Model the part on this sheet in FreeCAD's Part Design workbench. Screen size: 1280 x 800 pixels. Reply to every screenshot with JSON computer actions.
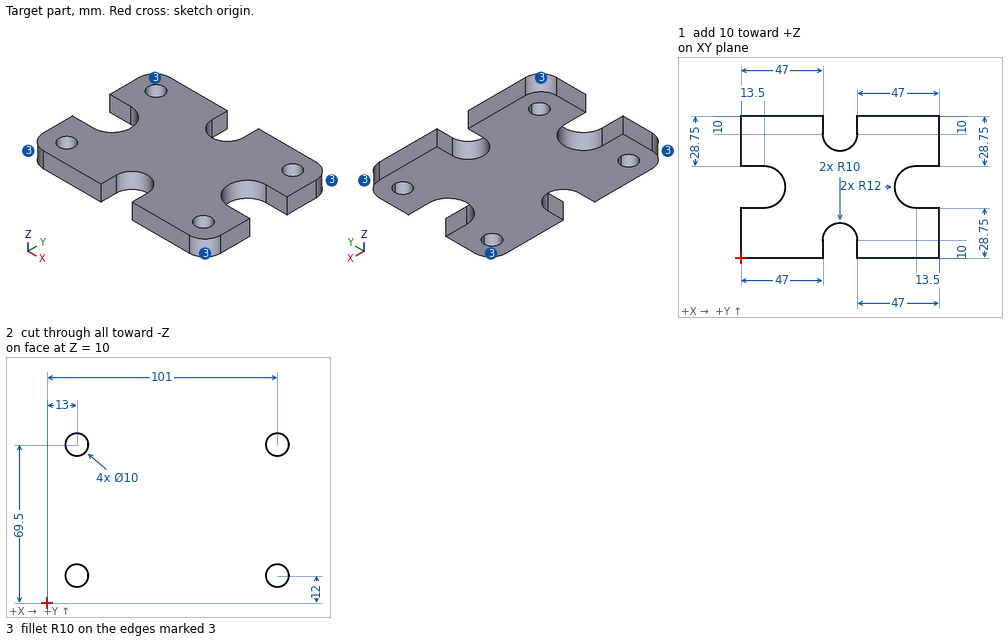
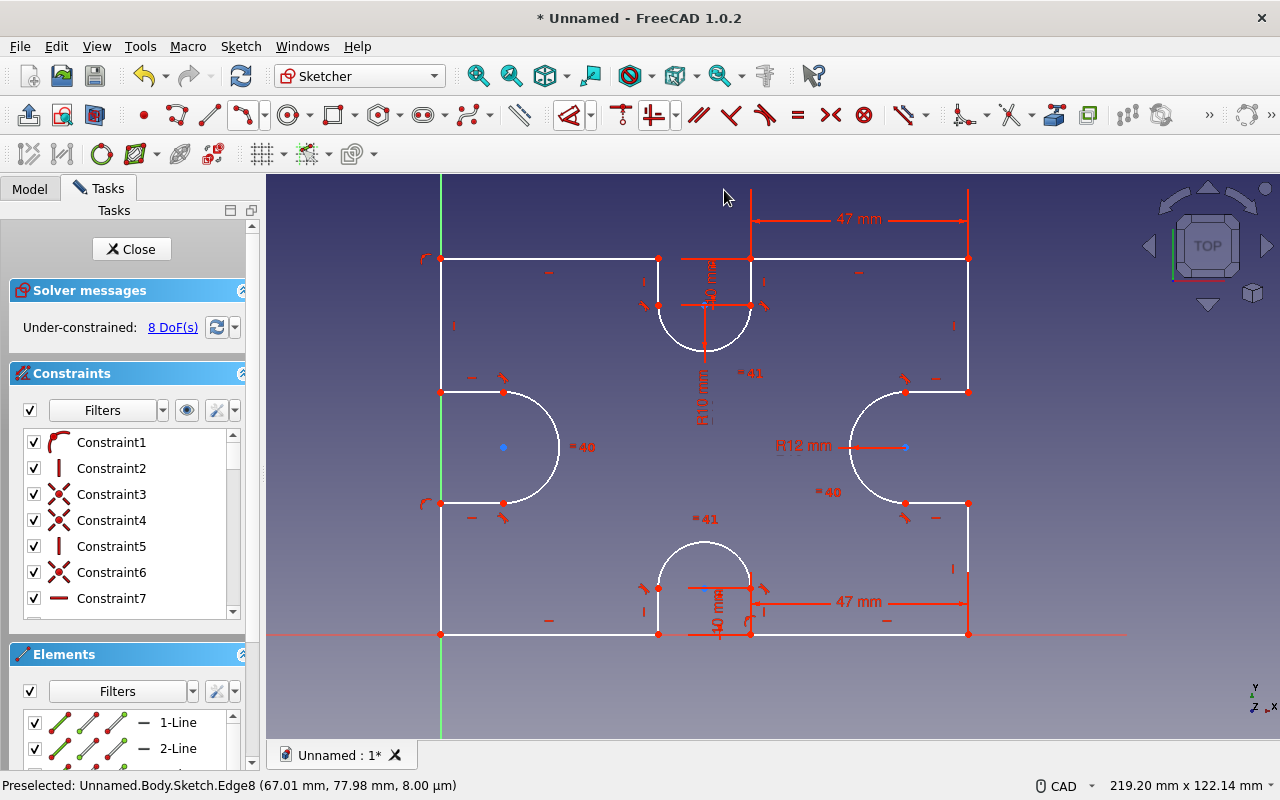
{"action": "left_click", "coordinate": [658, 291]}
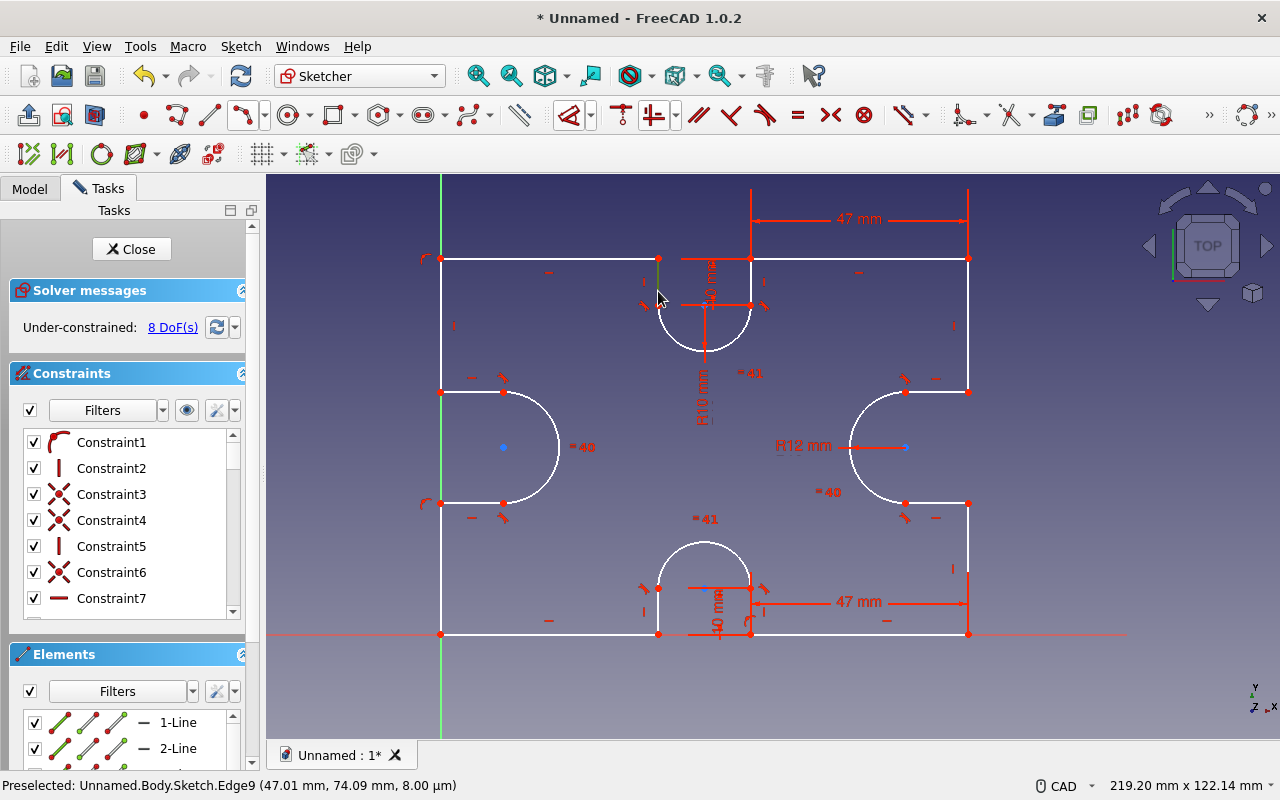
{"action": "key", "text": "i"}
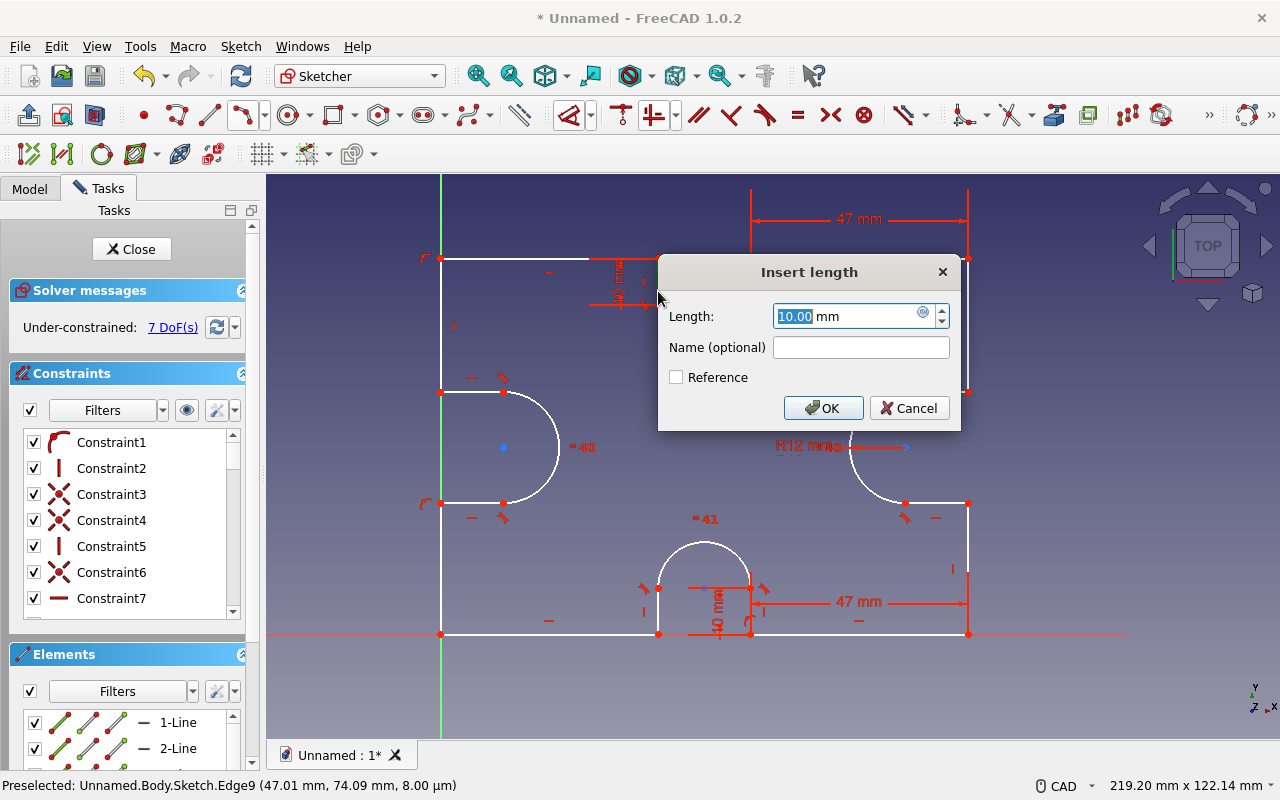
{"action": "type", "text": "10"}
{"action": "key", "text": "Return"}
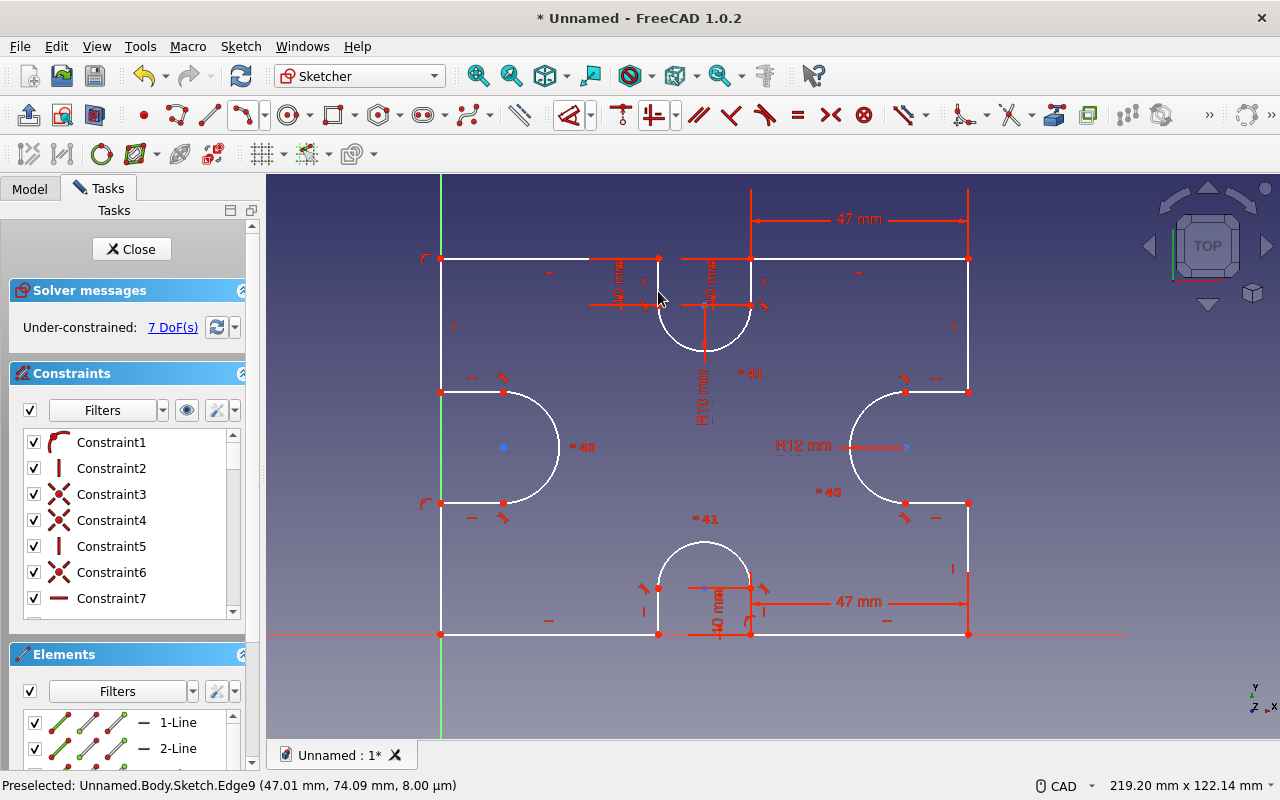
{"action": "left_click", "coordinate": [593, 259]}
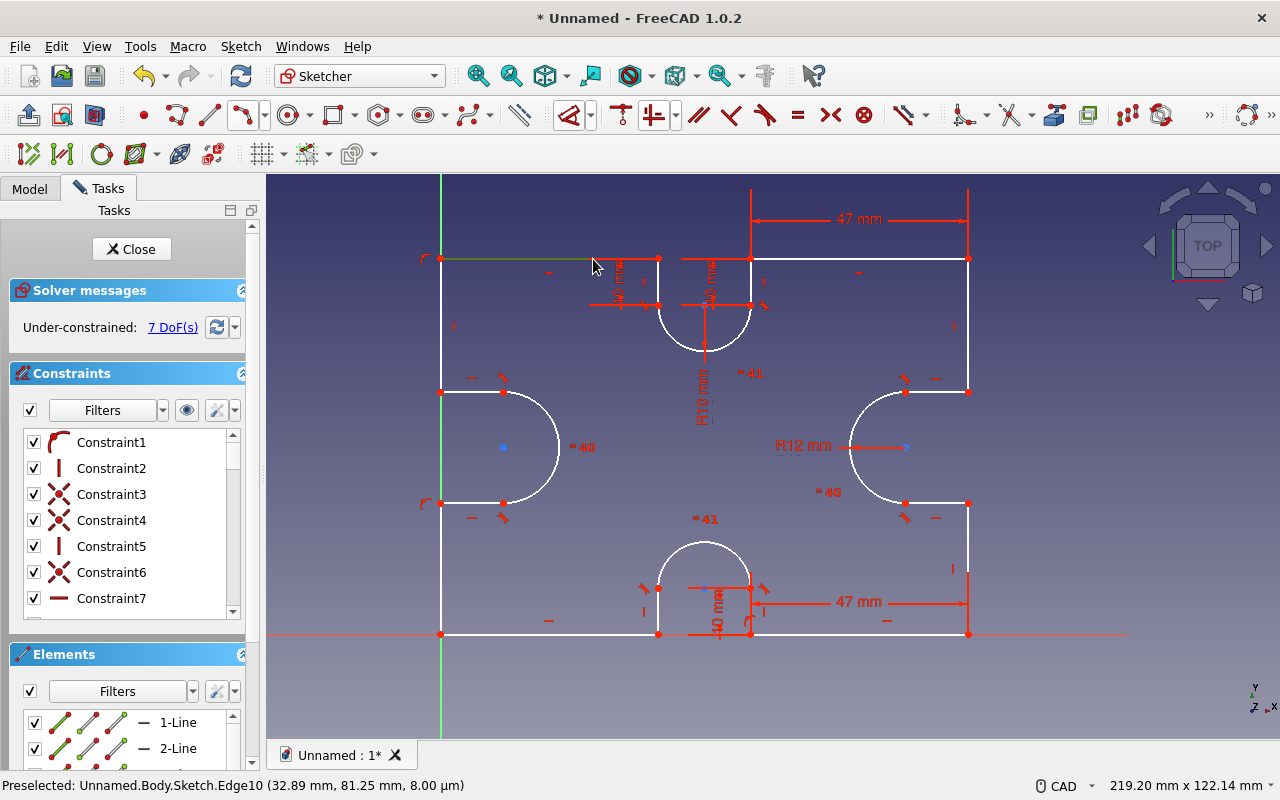
{"action": "left_click", "coordinate": [590, 116]}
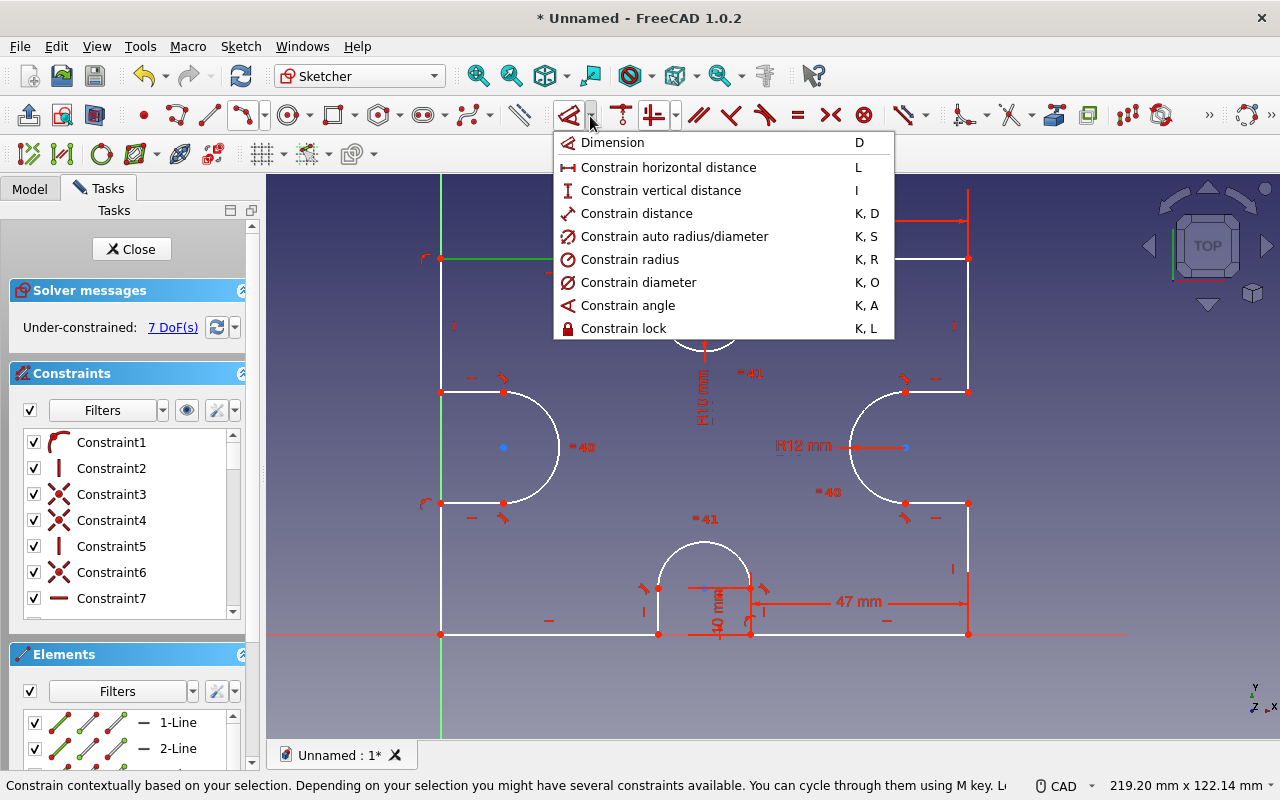
{"action": "left_click", "coordinate": [724, 168]}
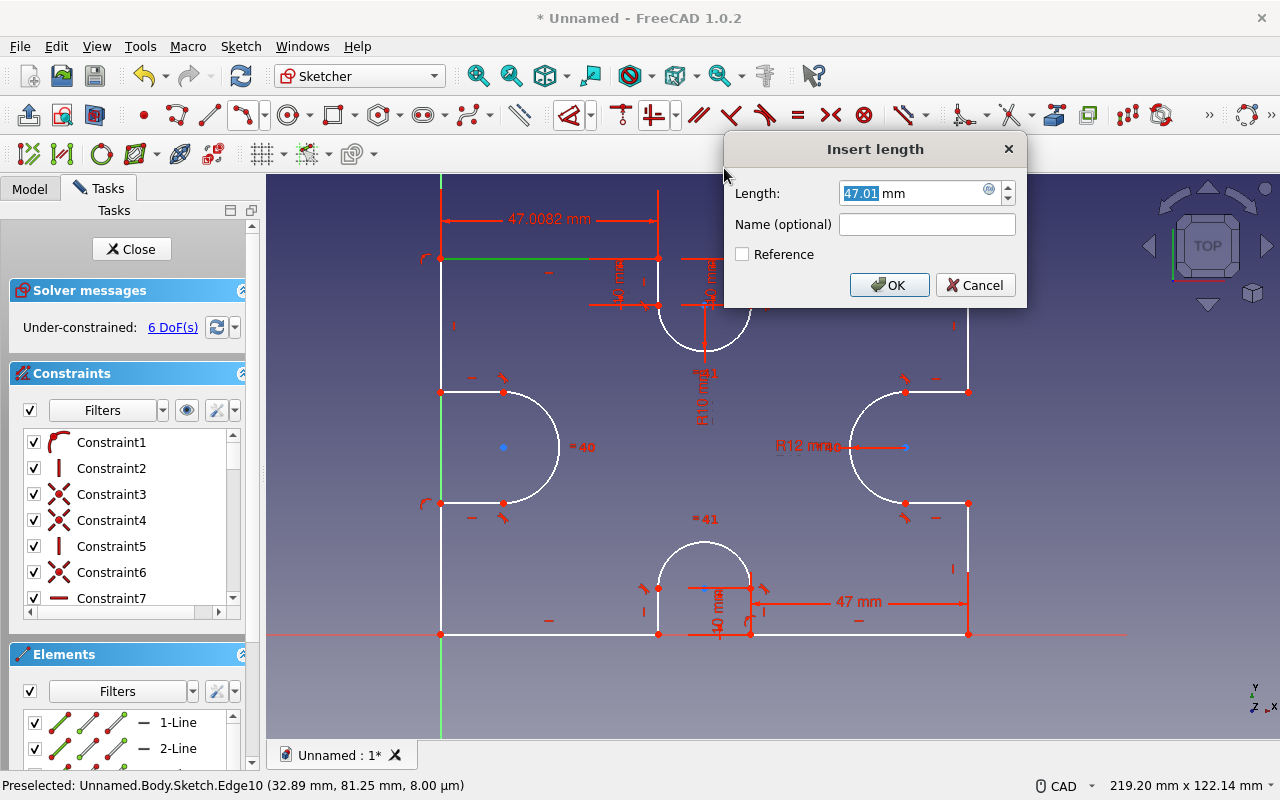
{"action": "type", "text": "47"}
{"action": "key", "text": "Return"}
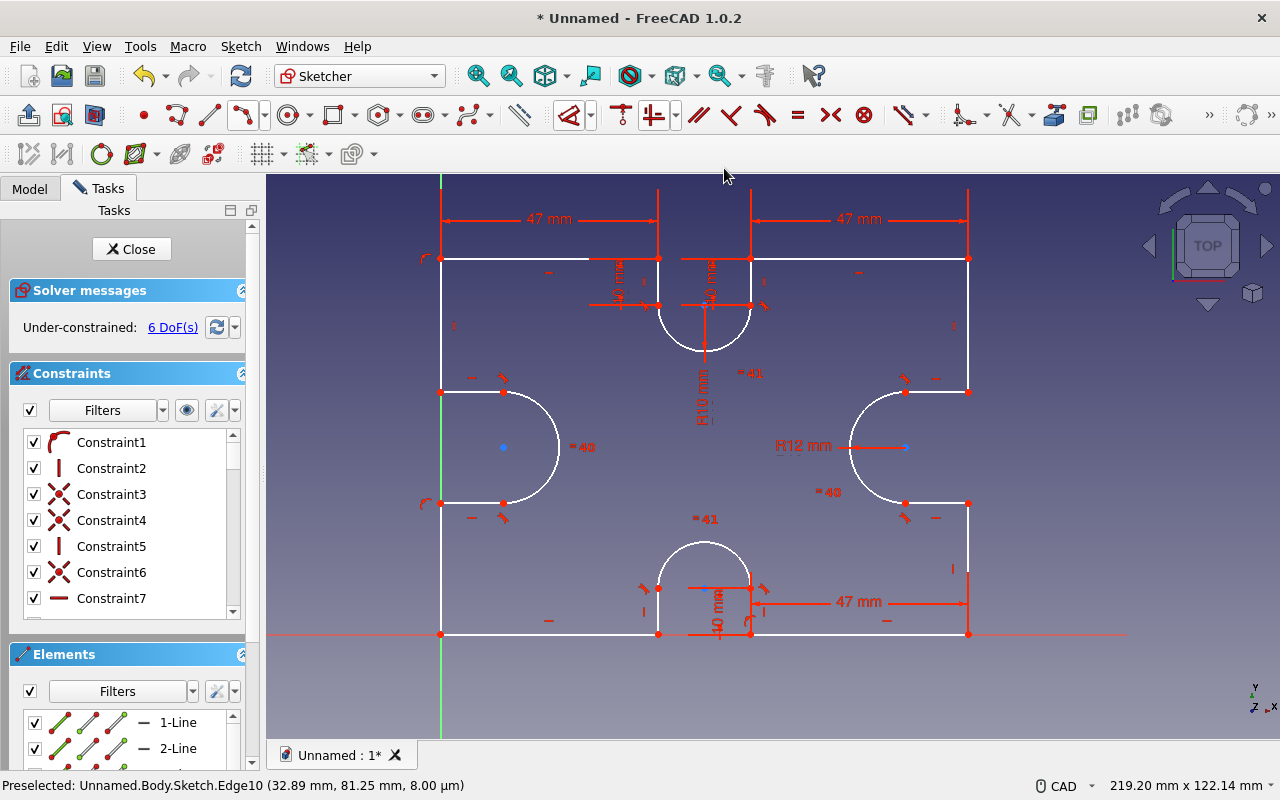
{"action": "left_click", "coordinate": [506, 635]}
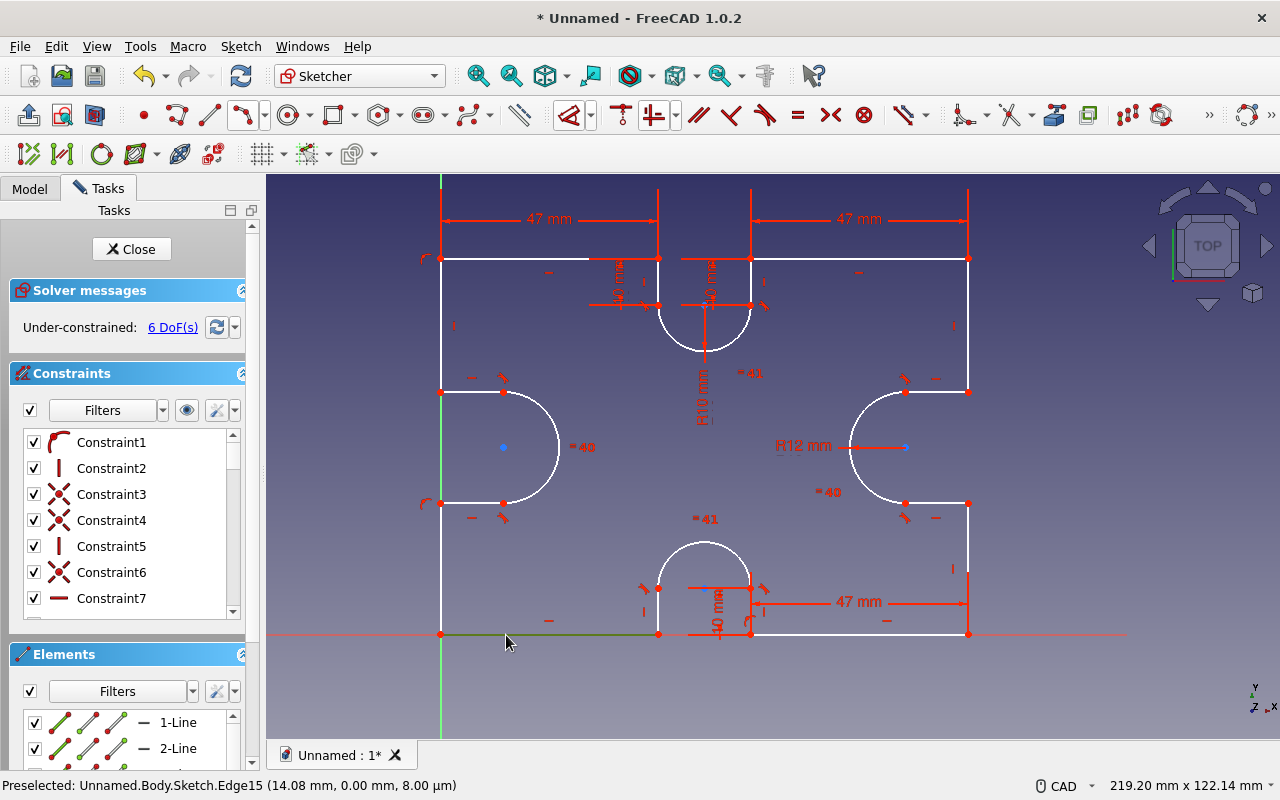
{"action": "key", "text": "l"}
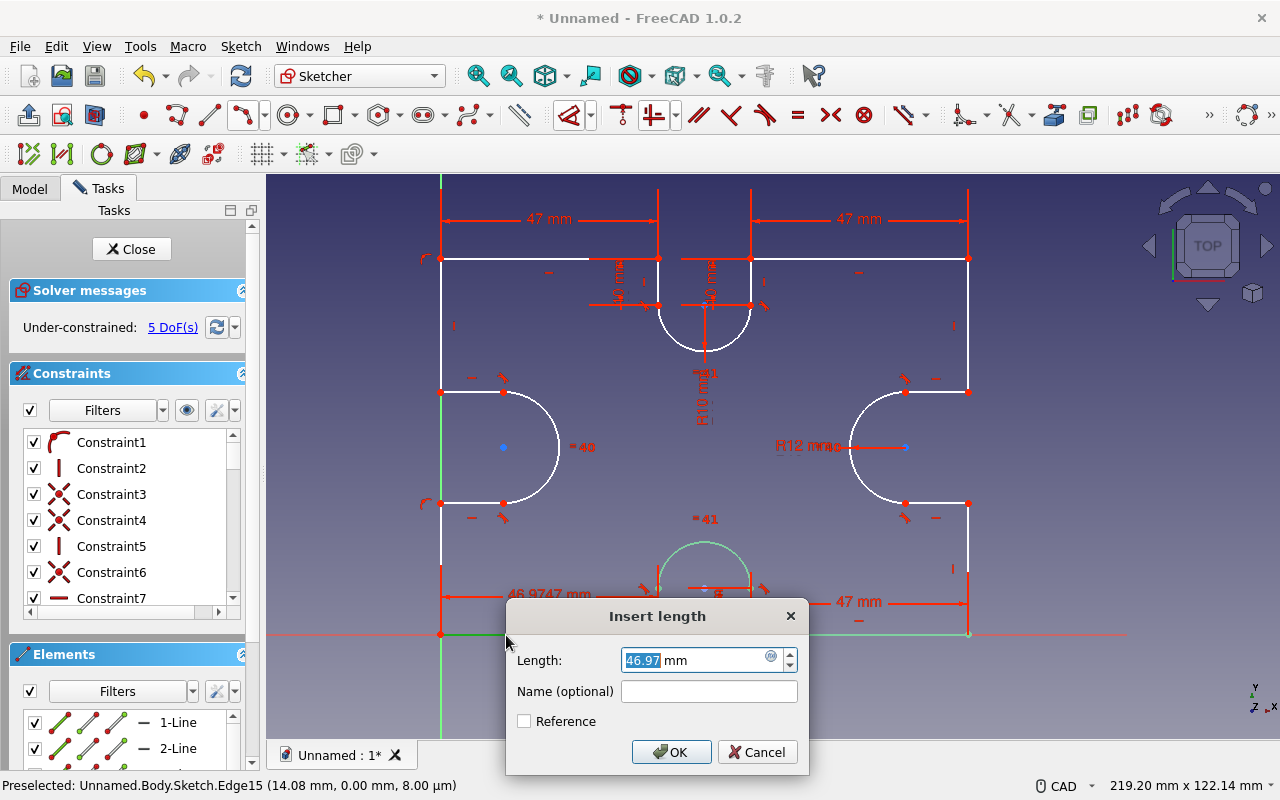
{"action": "type", "text": "47"}
{"action": "key", "text": "Return"}